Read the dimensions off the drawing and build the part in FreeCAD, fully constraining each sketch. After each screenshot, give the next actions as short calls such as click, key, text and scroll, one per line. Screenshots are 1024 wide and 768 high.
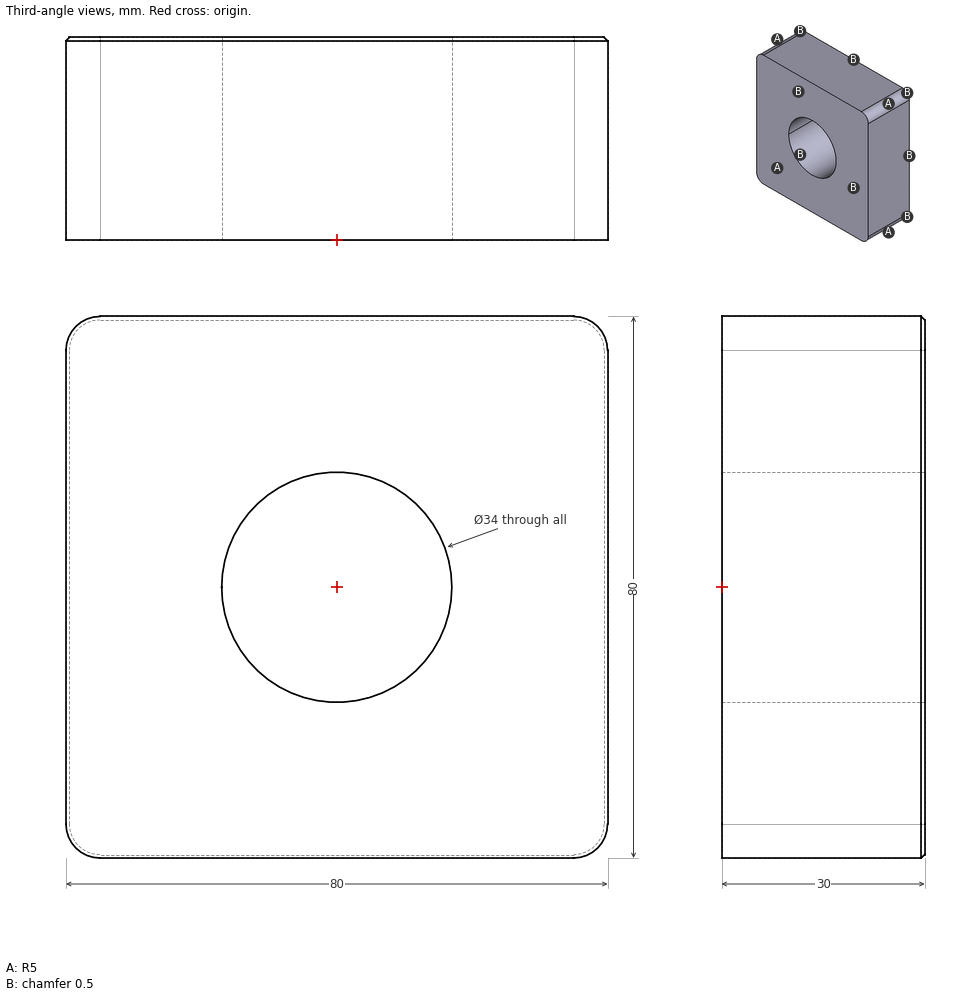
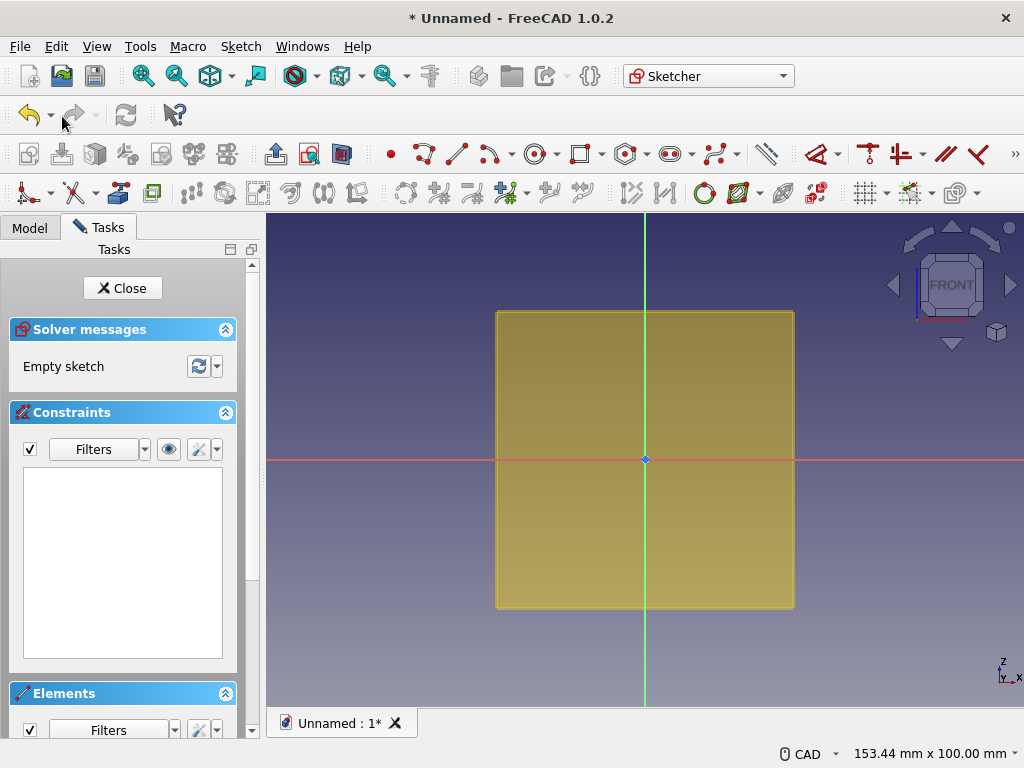
scroll(294, 460, down, 1)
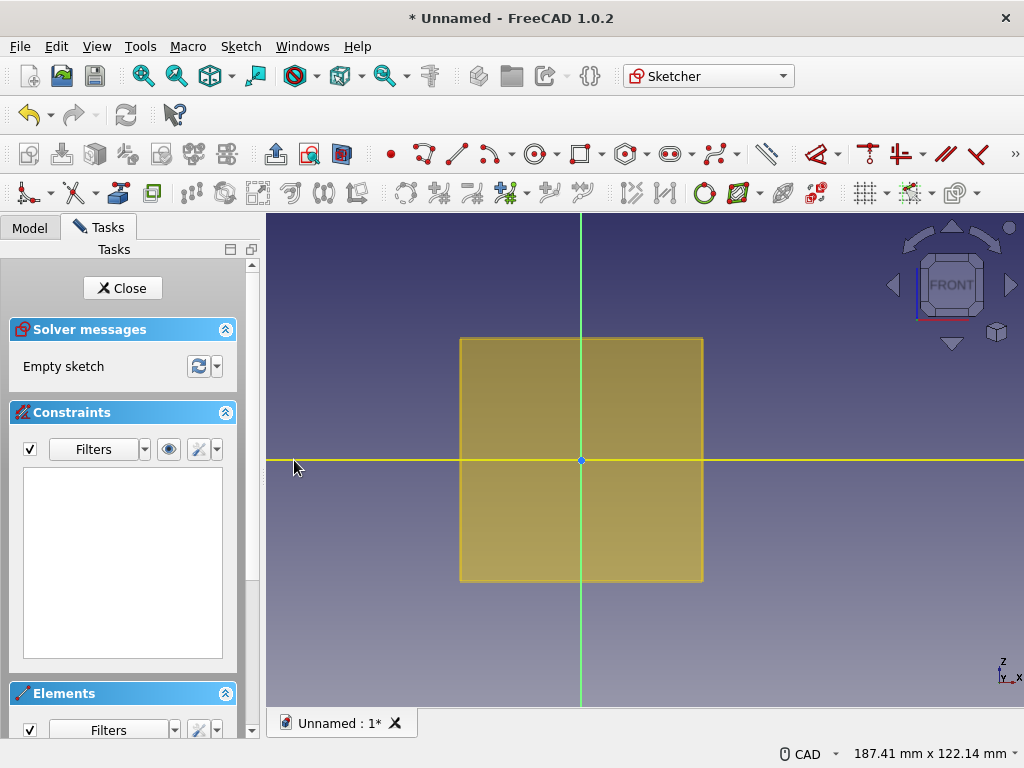
click(602, 154)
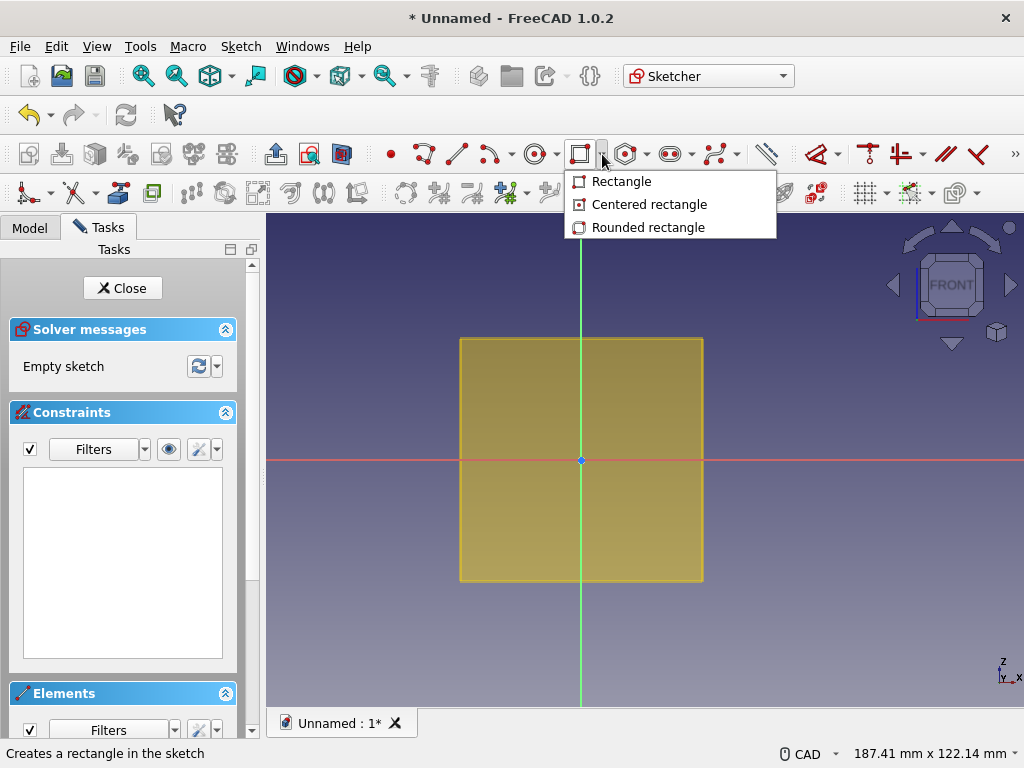
click(670, 204)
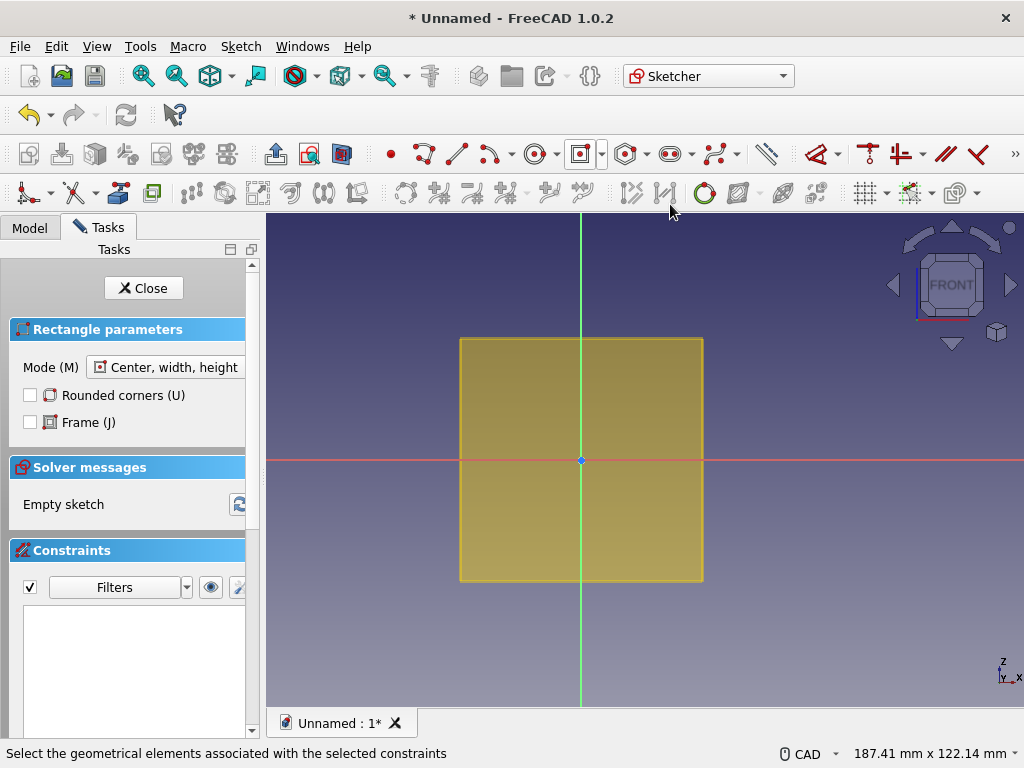
click(581, 460)
click(743, 298)
key(Escape)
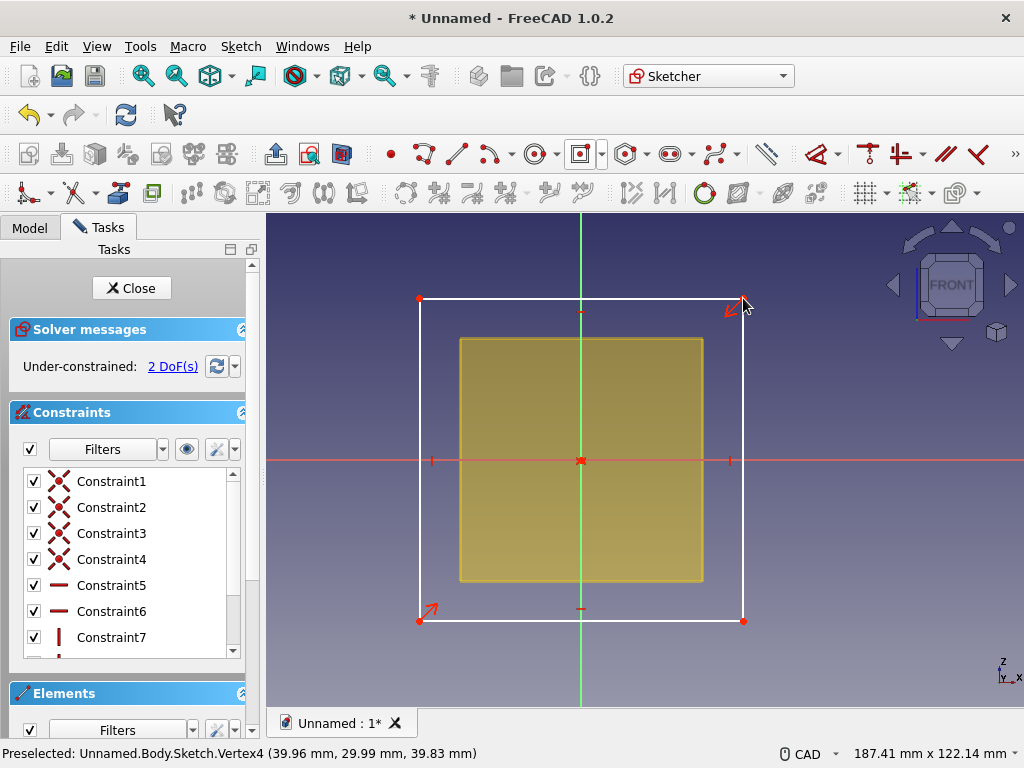
click(517, 621)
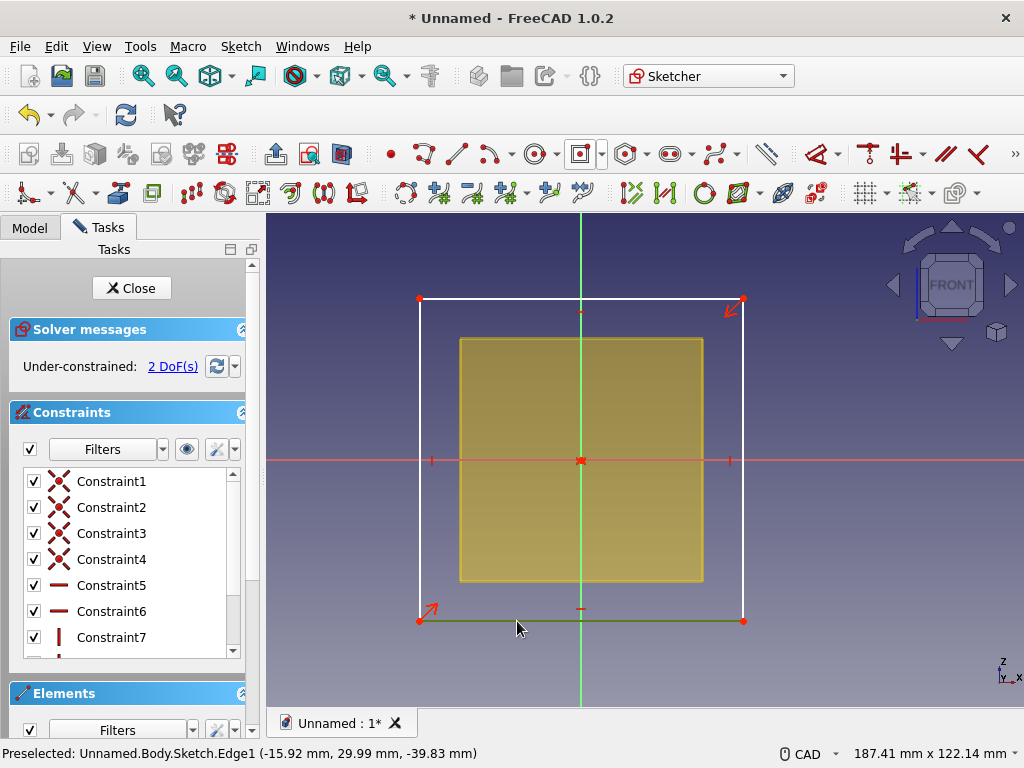
key(l)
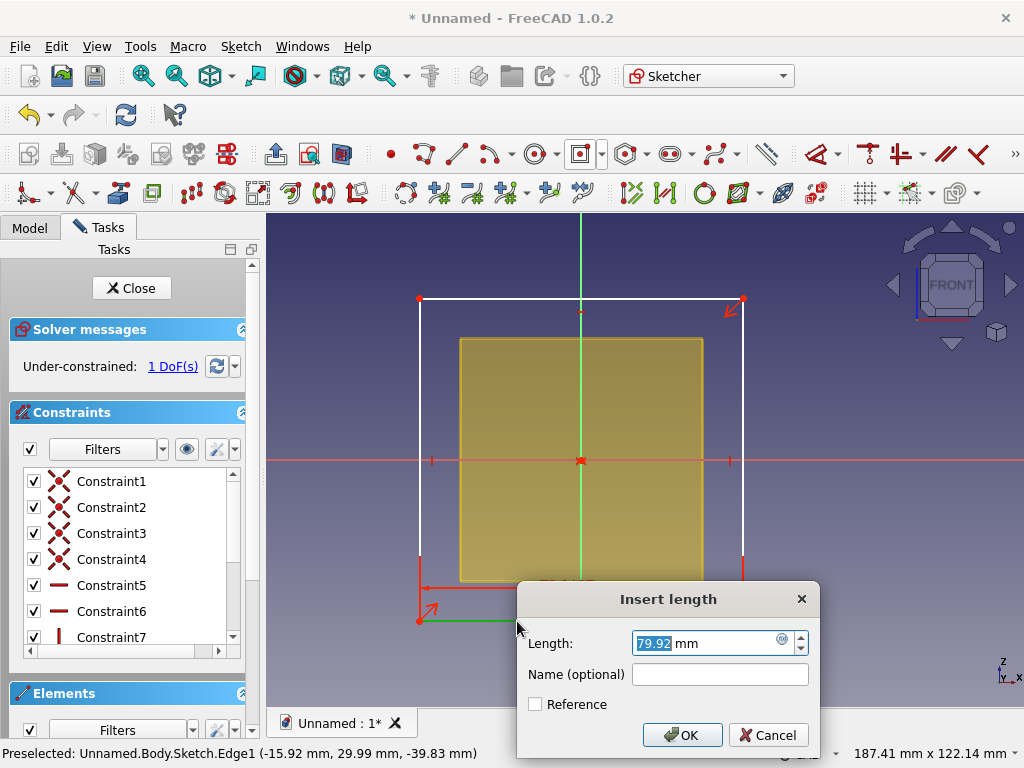
text(80)
key(Return)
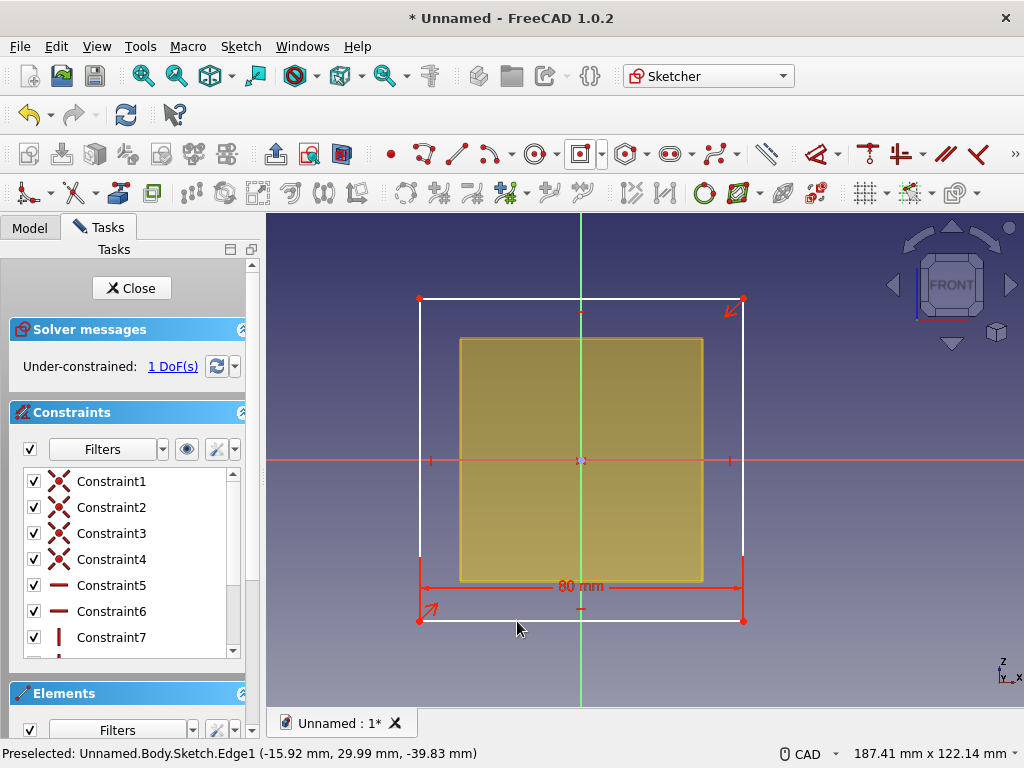
click(743, 525)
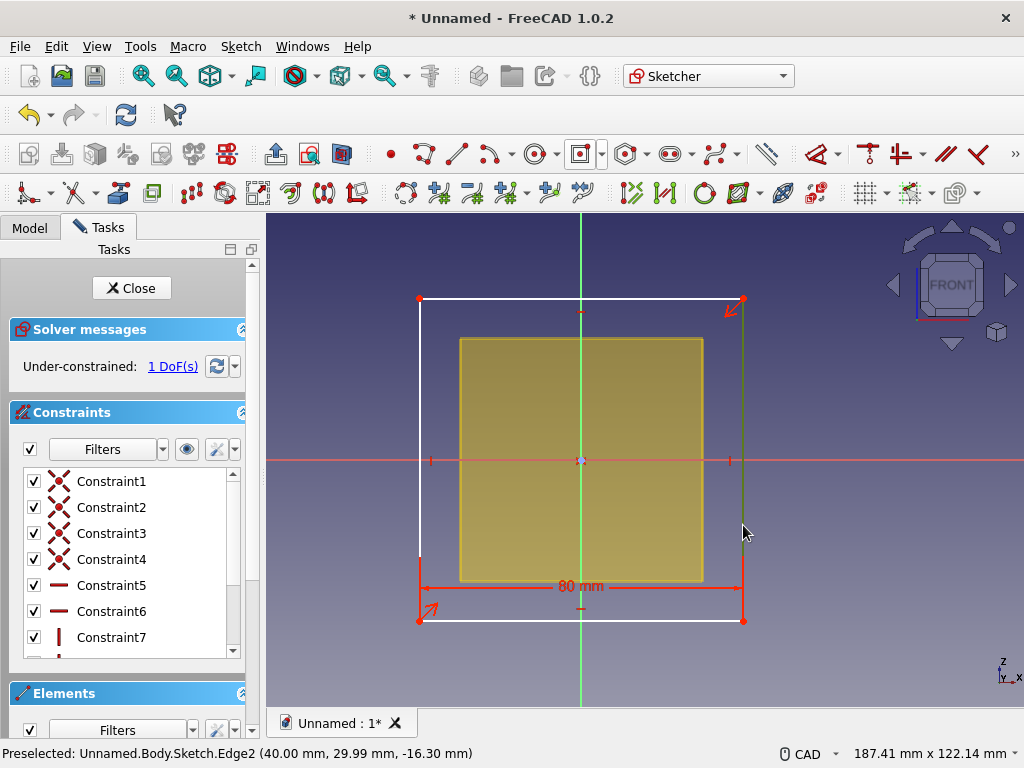
click(838, 154)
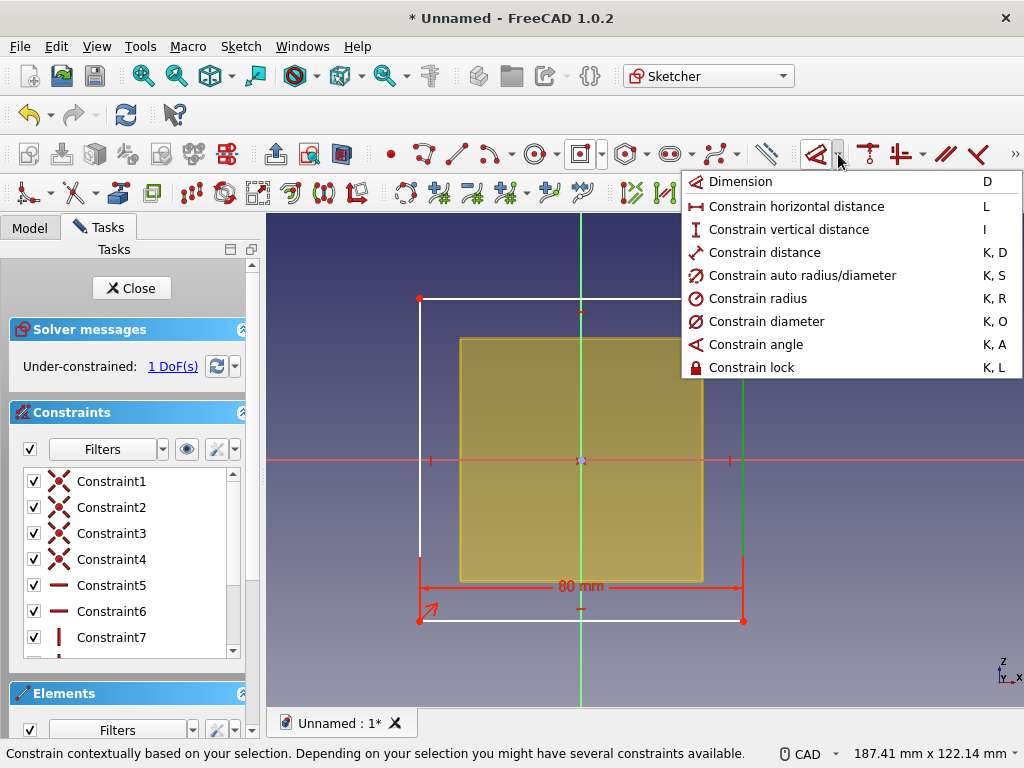
click(852, 230)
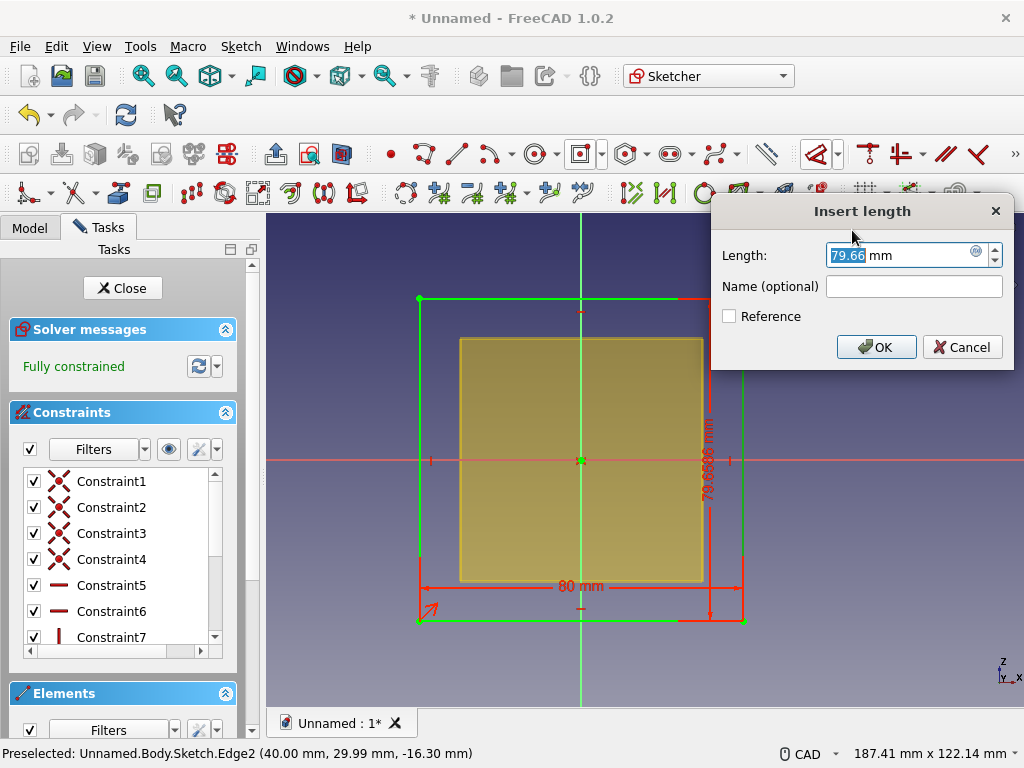
text(80)
key(Return)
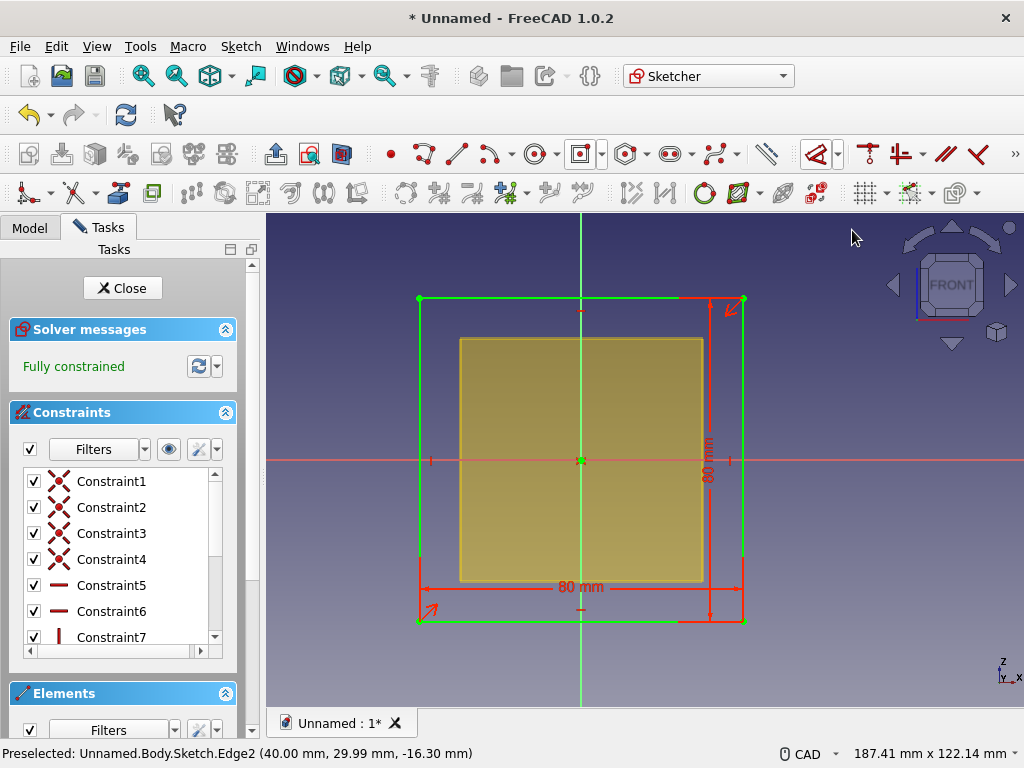
click(123, 288)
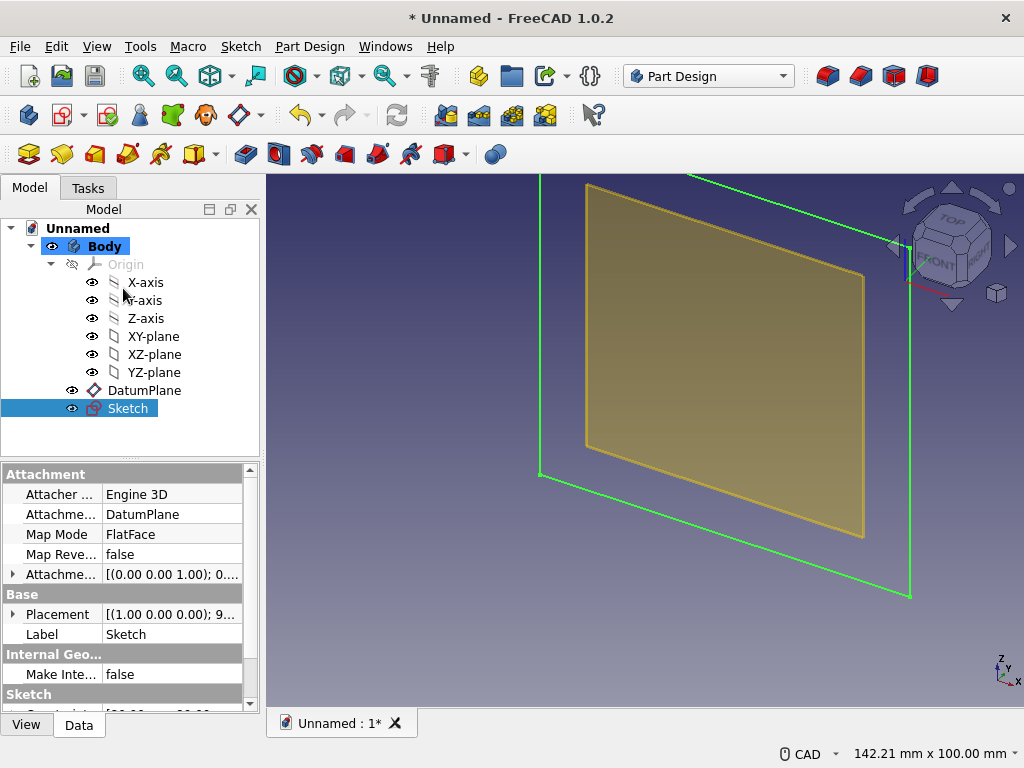
click(29, 154)